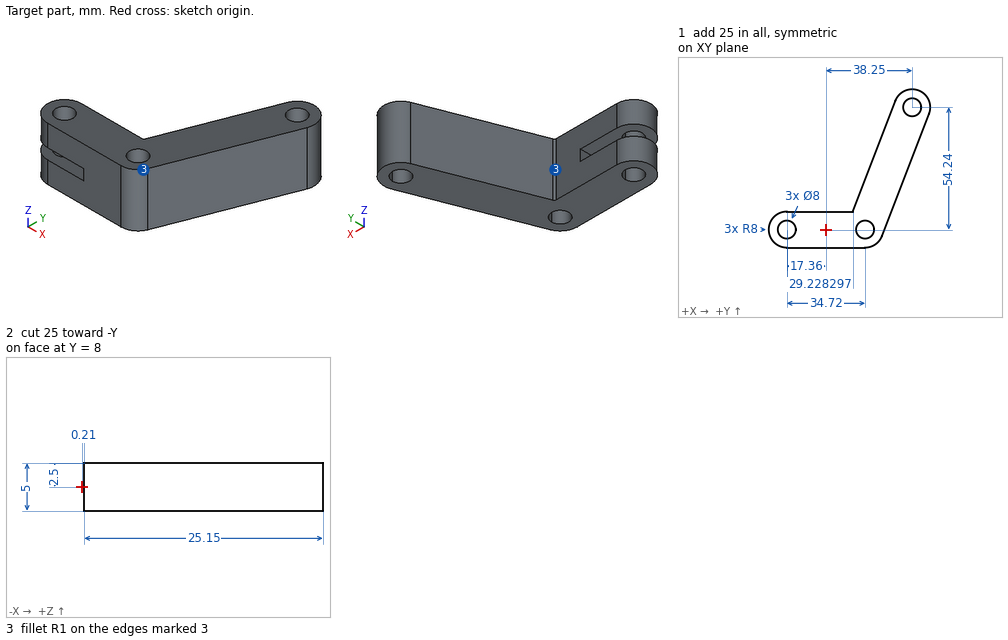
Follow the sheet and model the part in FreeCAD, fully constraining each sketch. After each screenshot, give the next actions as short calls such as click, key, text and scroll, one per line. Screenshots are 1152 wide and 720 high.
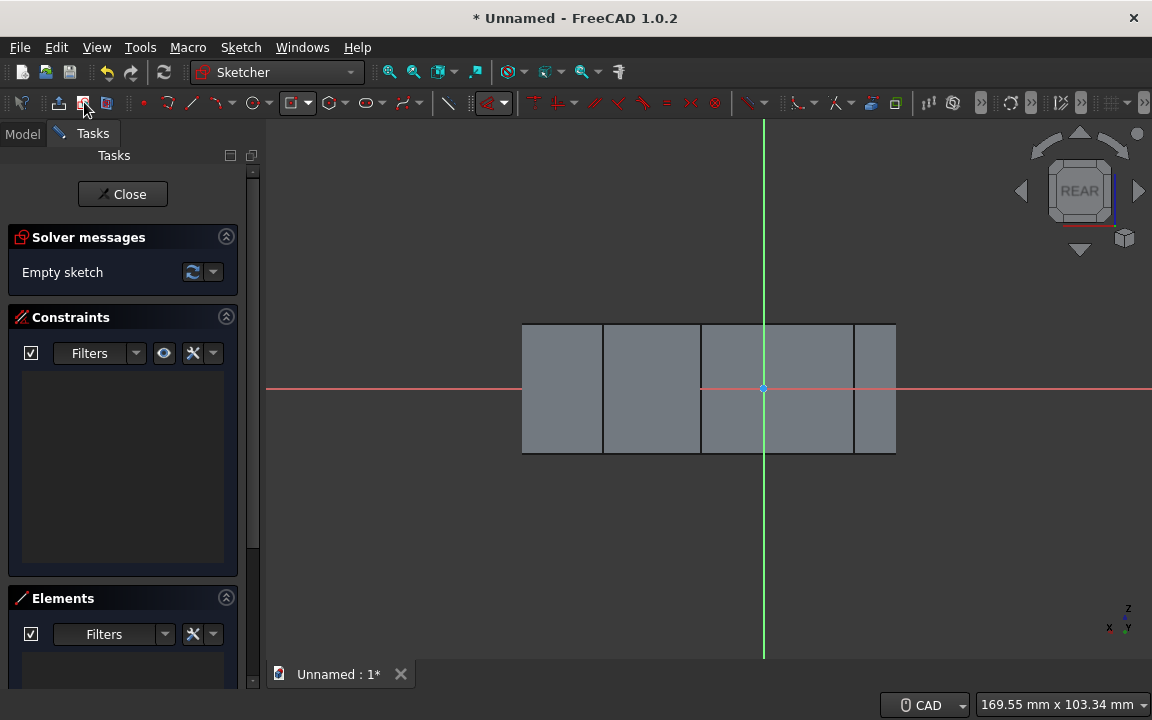
scroll(892, 389, up, 7)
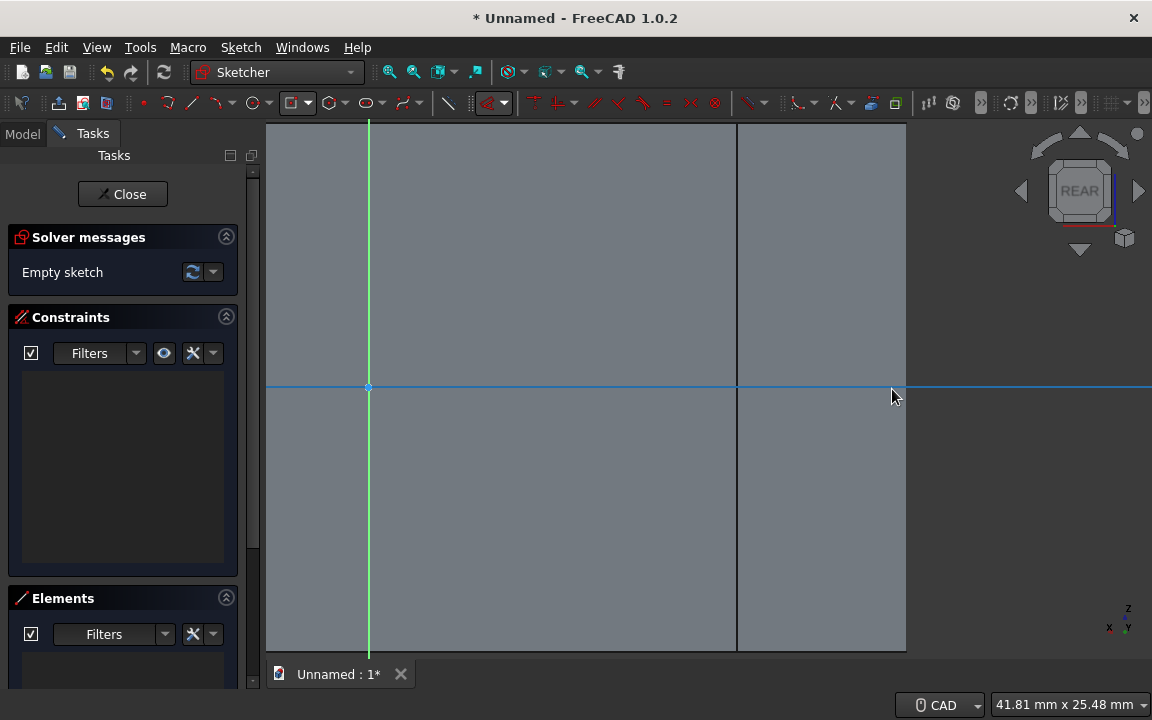
key(g)
key(r)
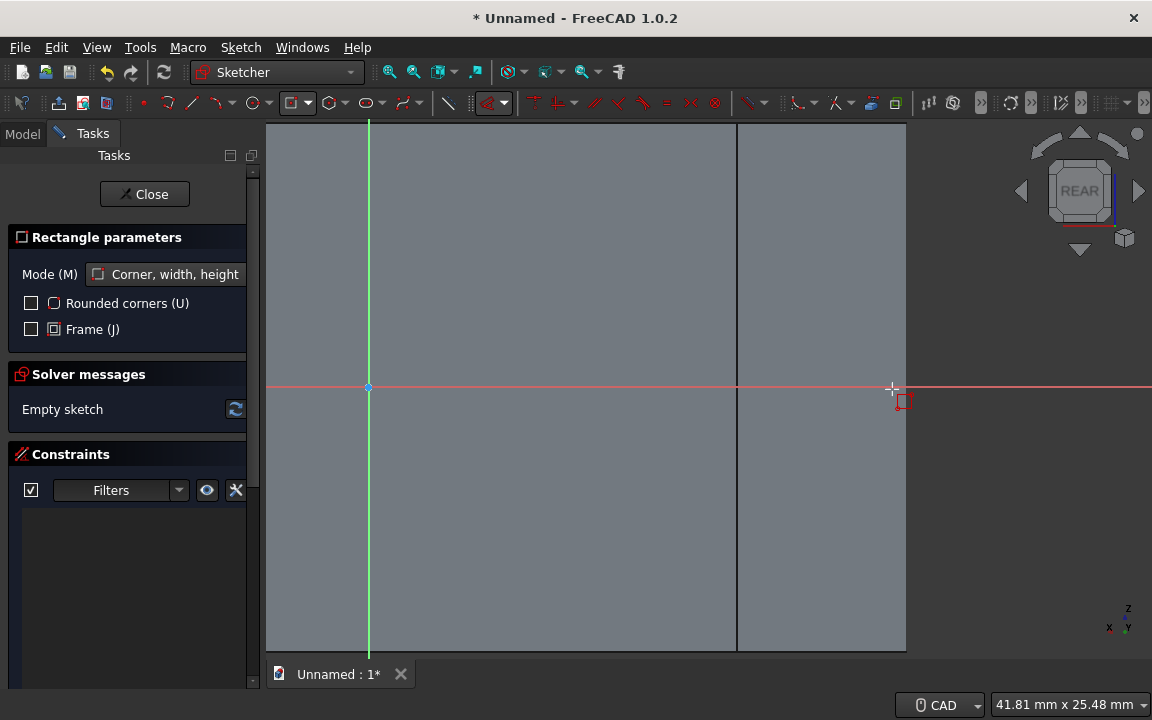
scroll(373, 334, up, 7)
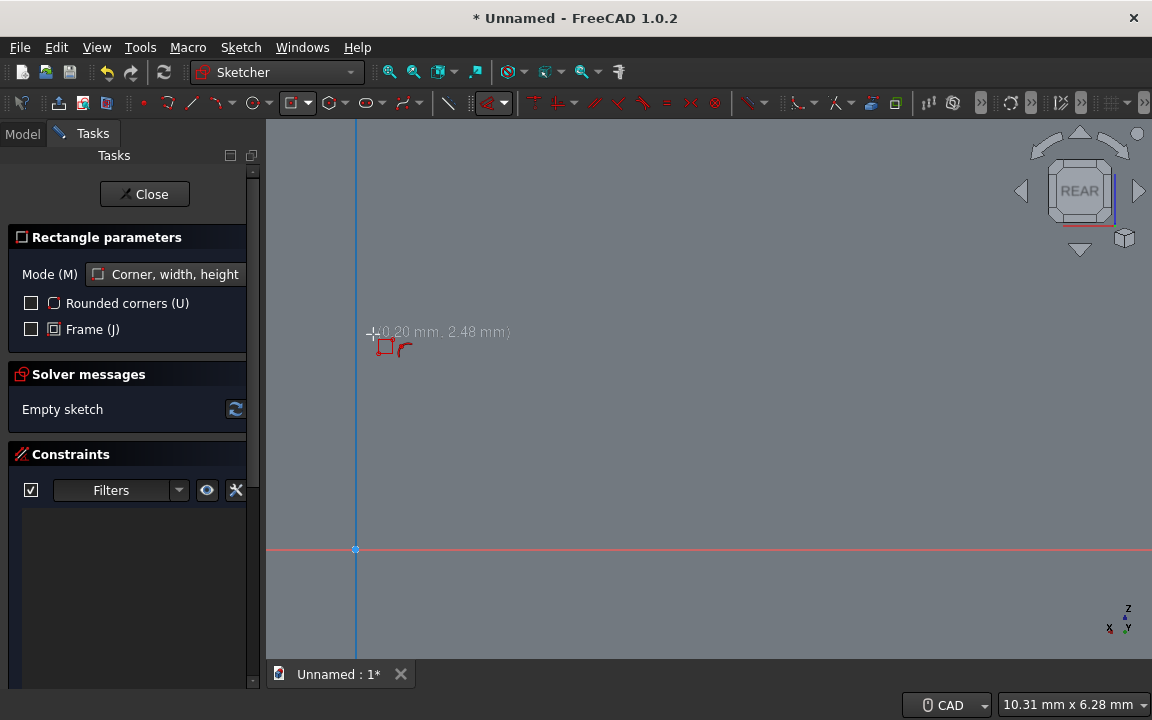
click(374, 335)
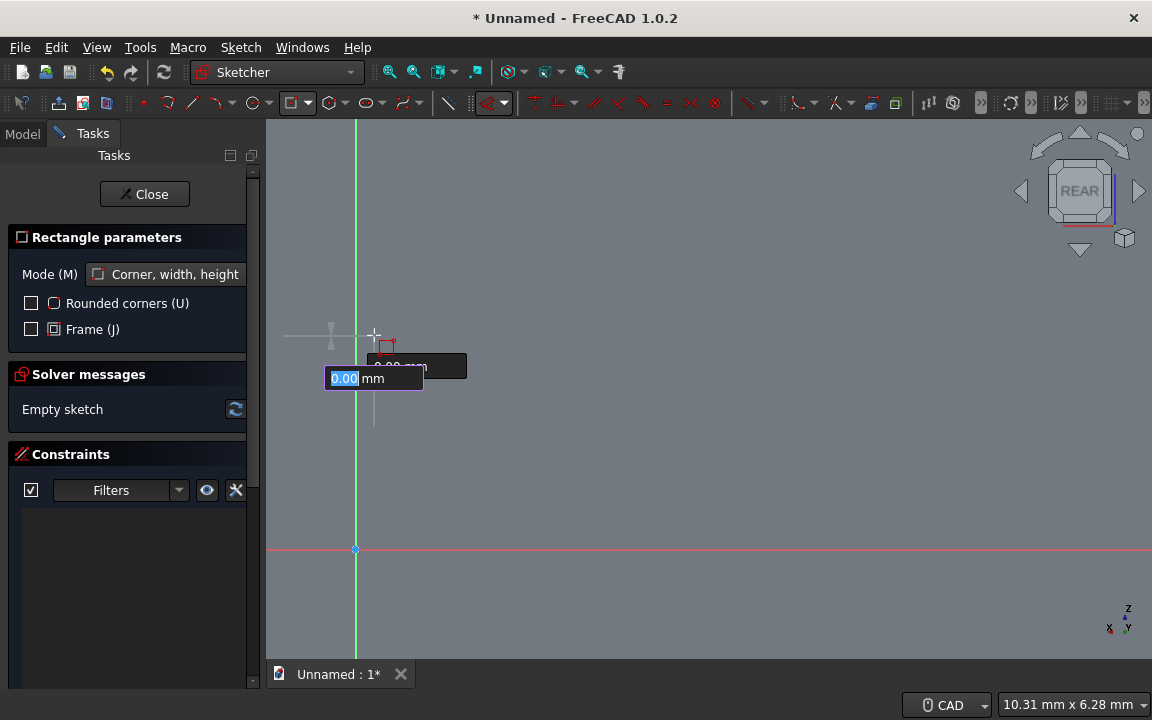
scroll(377, 336, down, 7)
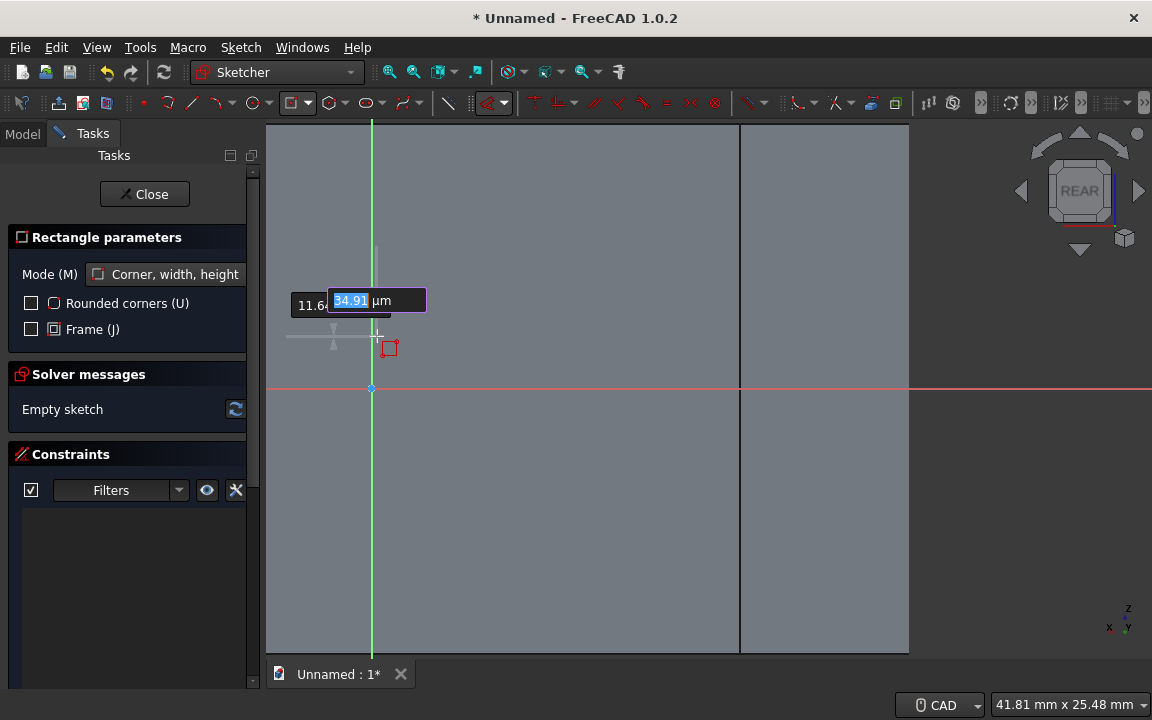
click(909, 442)
key(Escape)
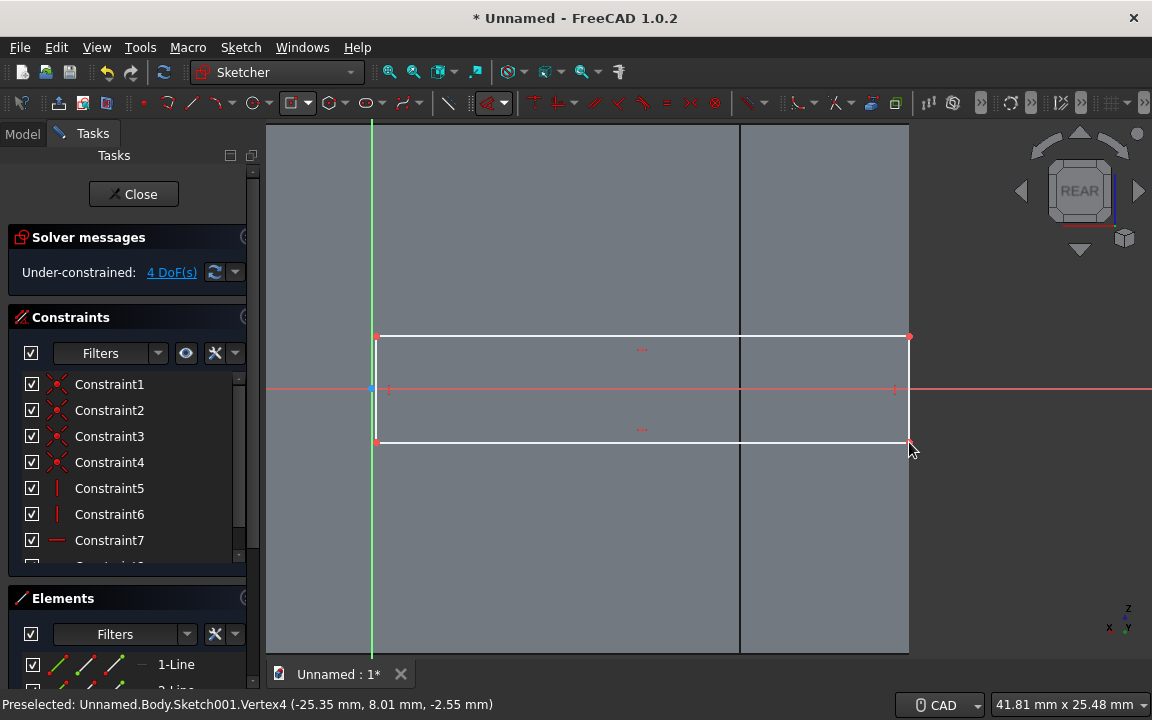
scroll(376, 368, up, 6)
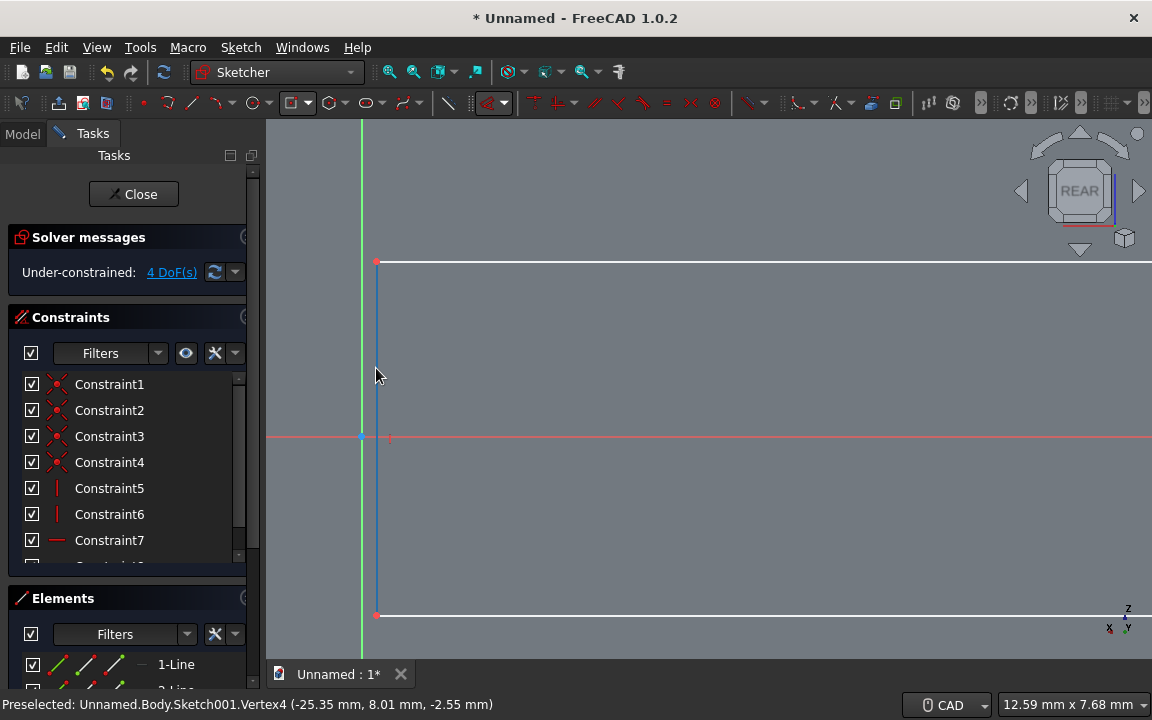
click(377, 368)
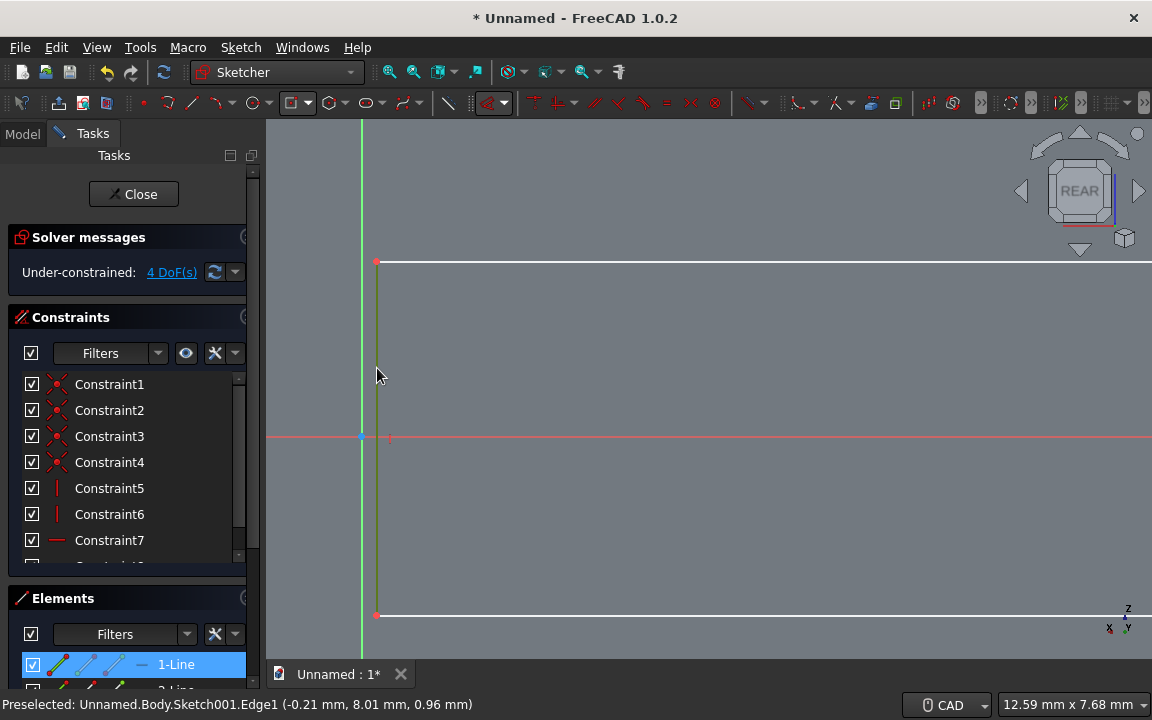
key(i)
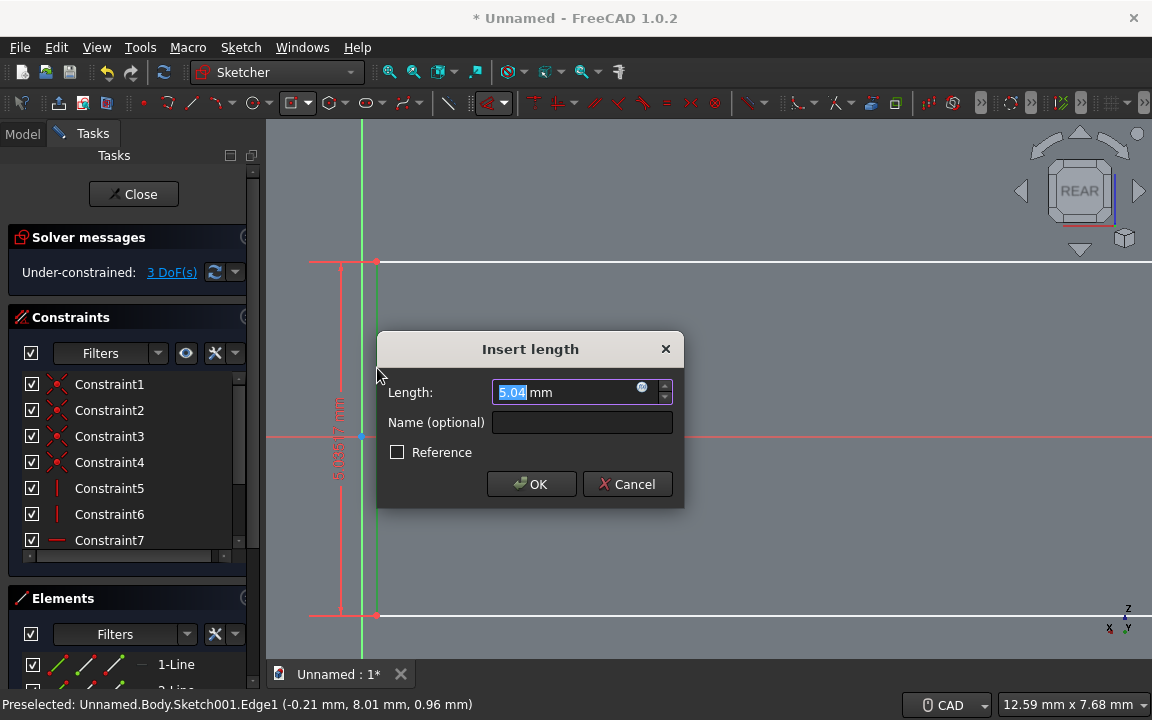
text(5)
key(Return)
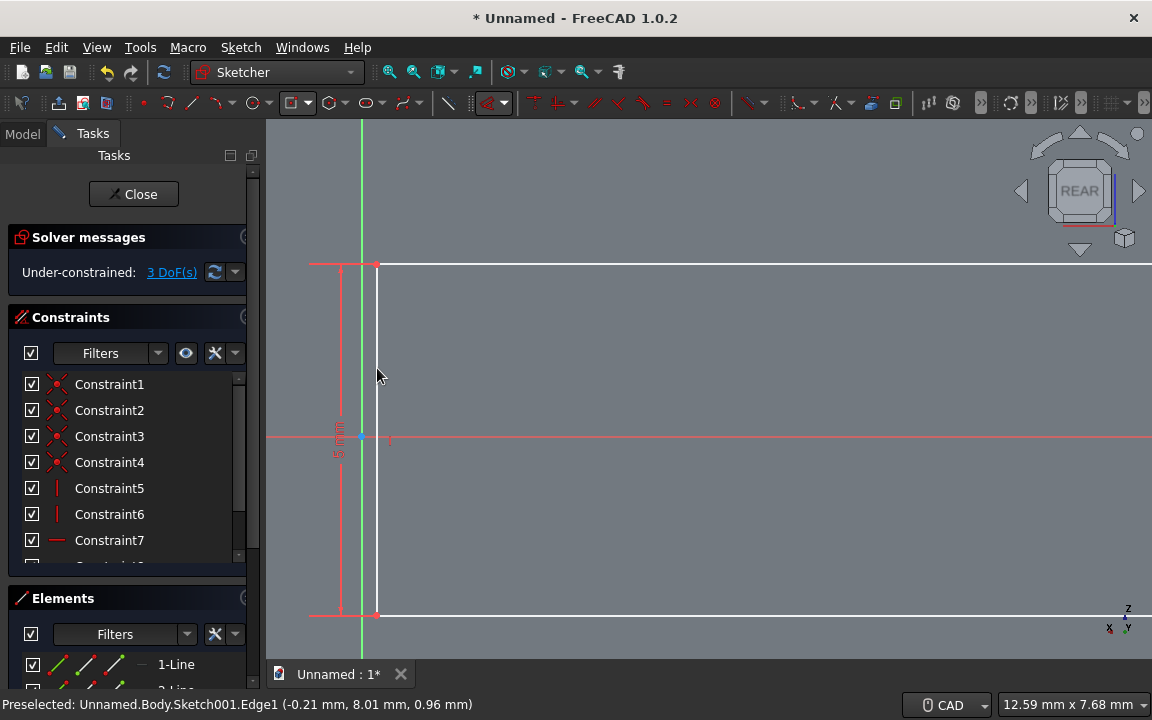
click(377, 264)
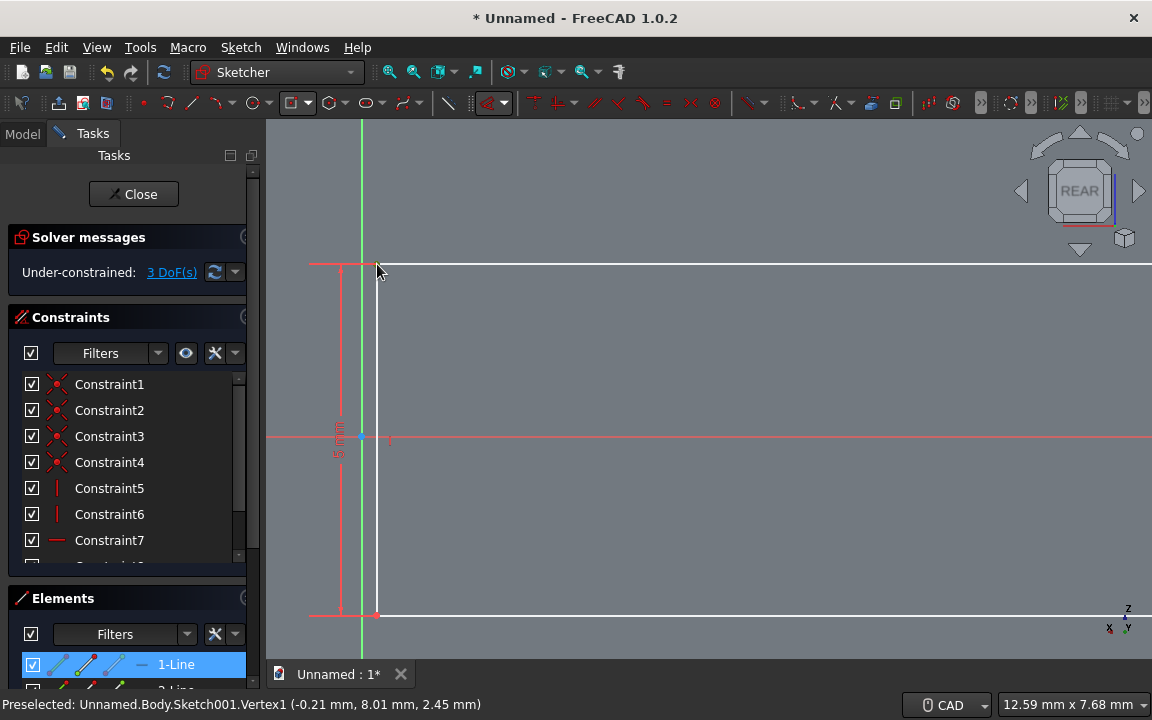
key(i)